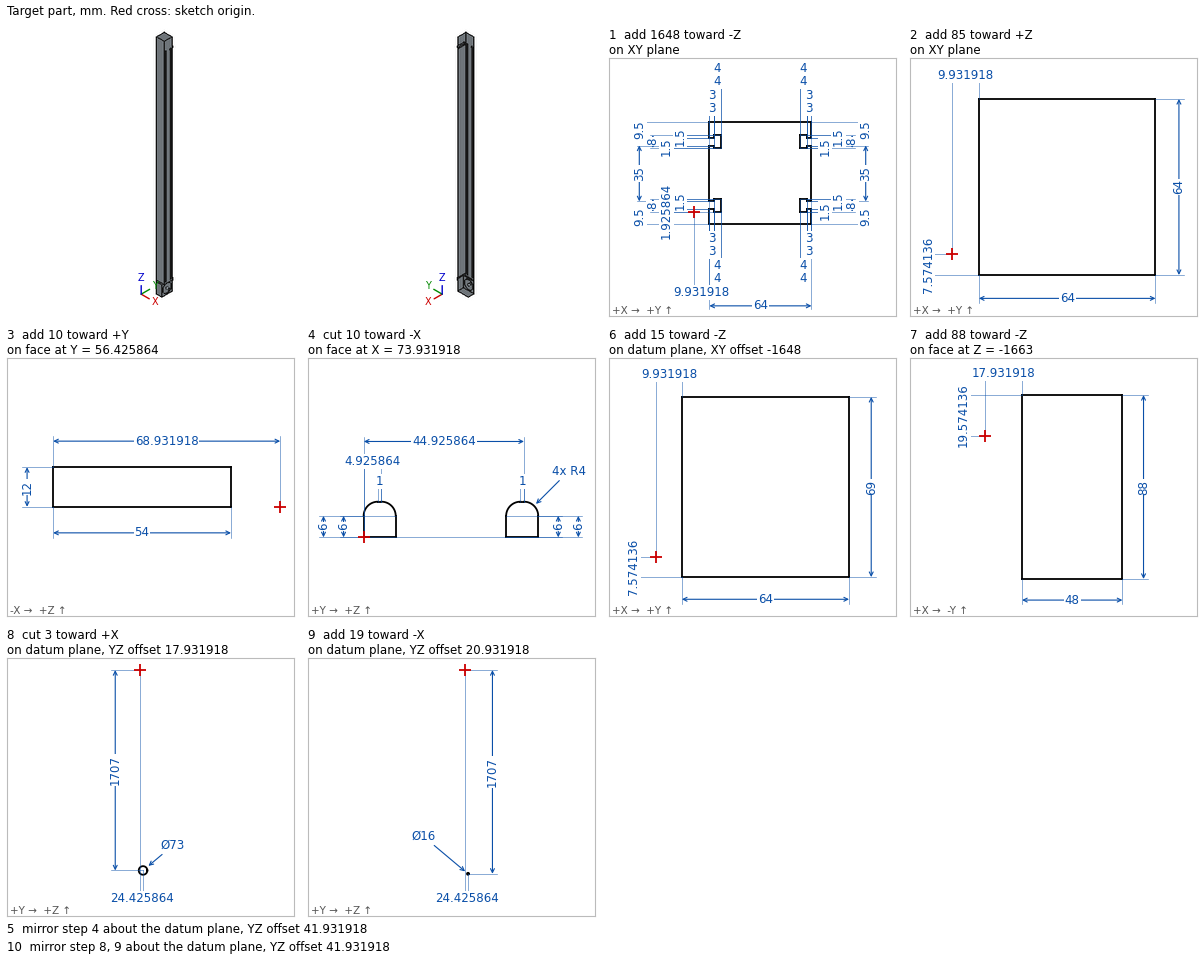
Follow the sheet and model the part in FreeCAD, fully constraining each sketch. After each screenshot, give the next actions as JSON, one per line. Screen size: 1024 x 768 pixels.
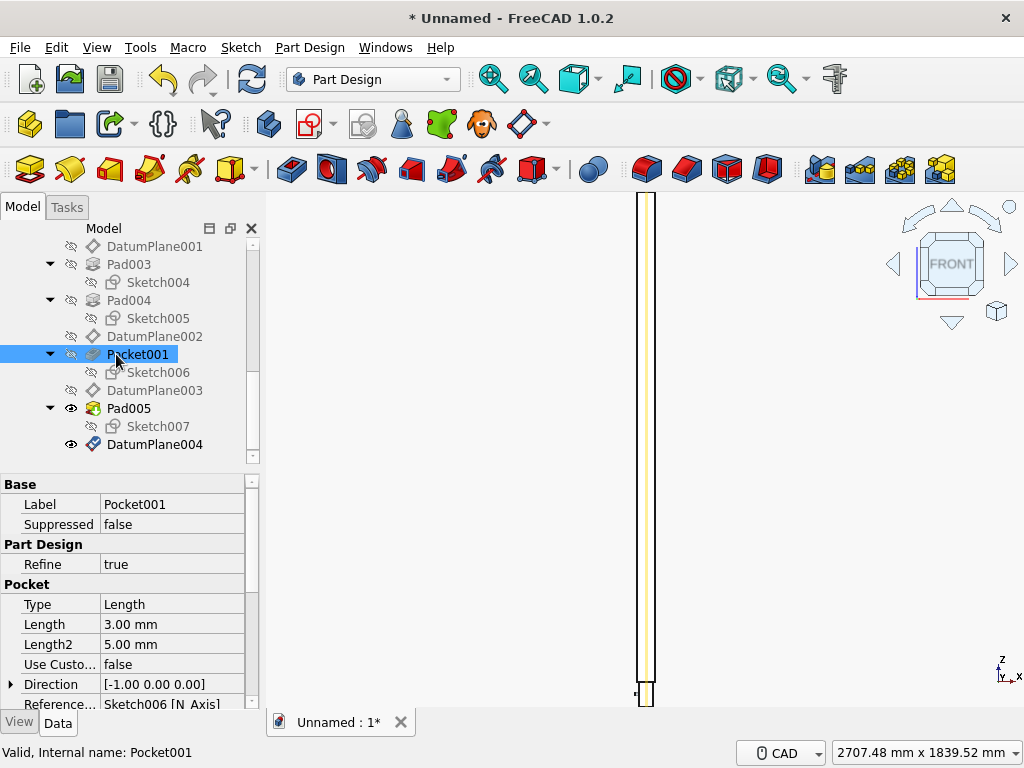
{"action": "left_click", "coordinate": [116, 408], "text": "ctrl"}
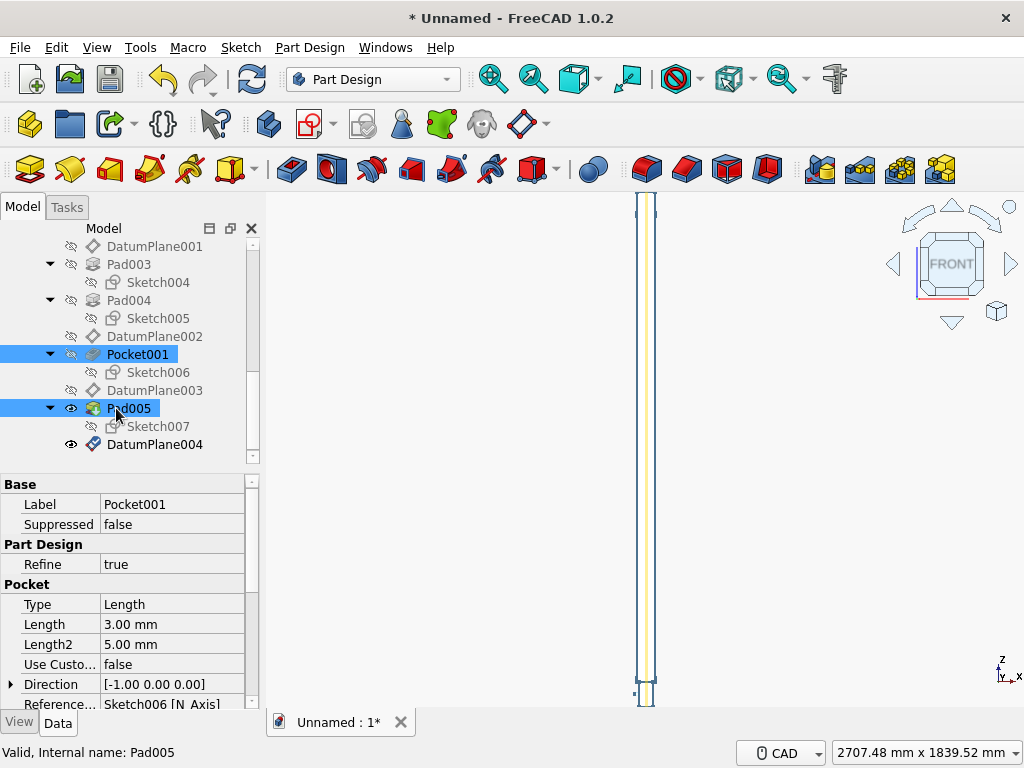
{"action": "left_click", "coordinate": [820, 170]}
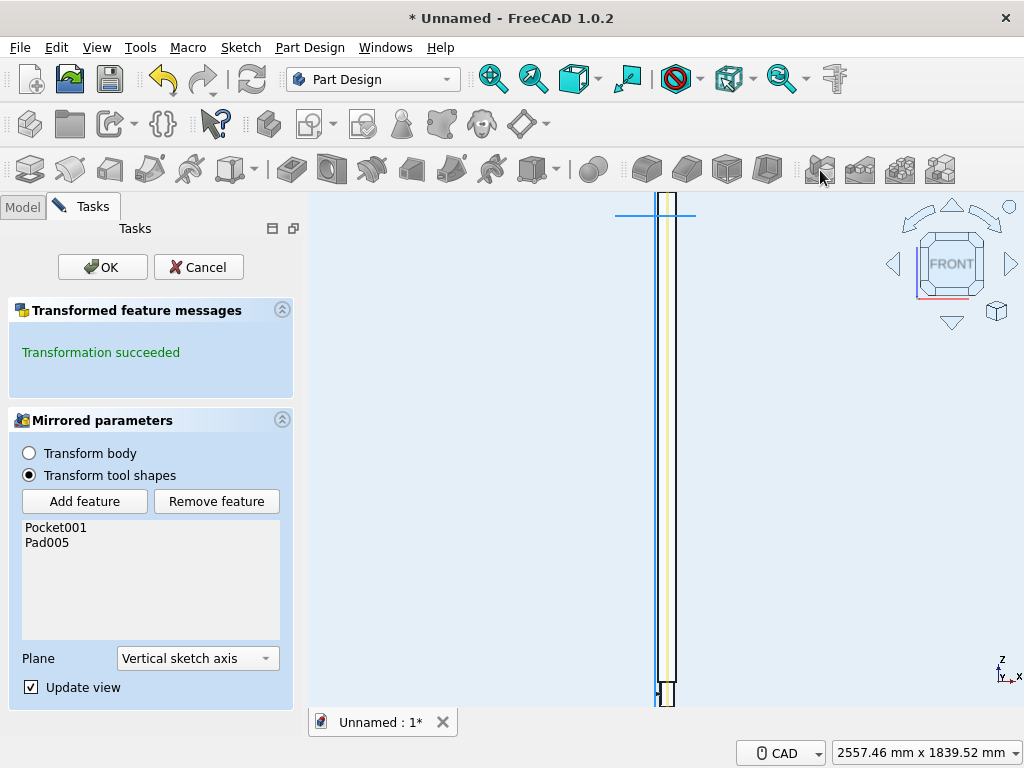
{"action": "left_click", "coordinate": [198, 658]}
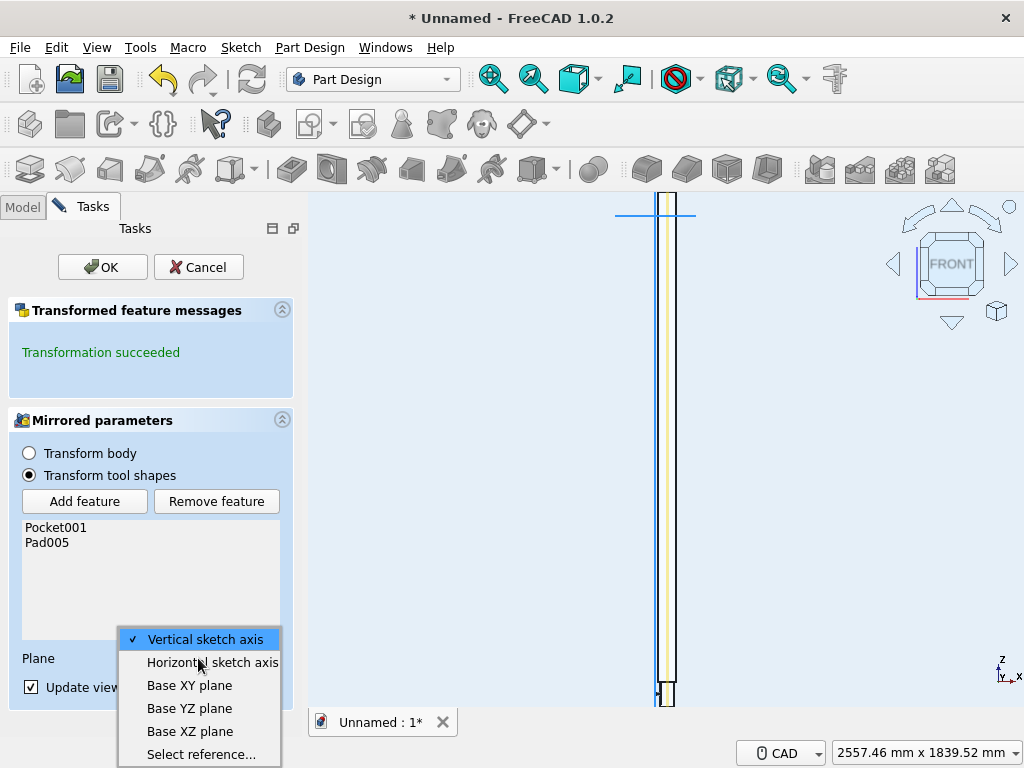
{"action": "left_click", "coordinate": [198, 754]}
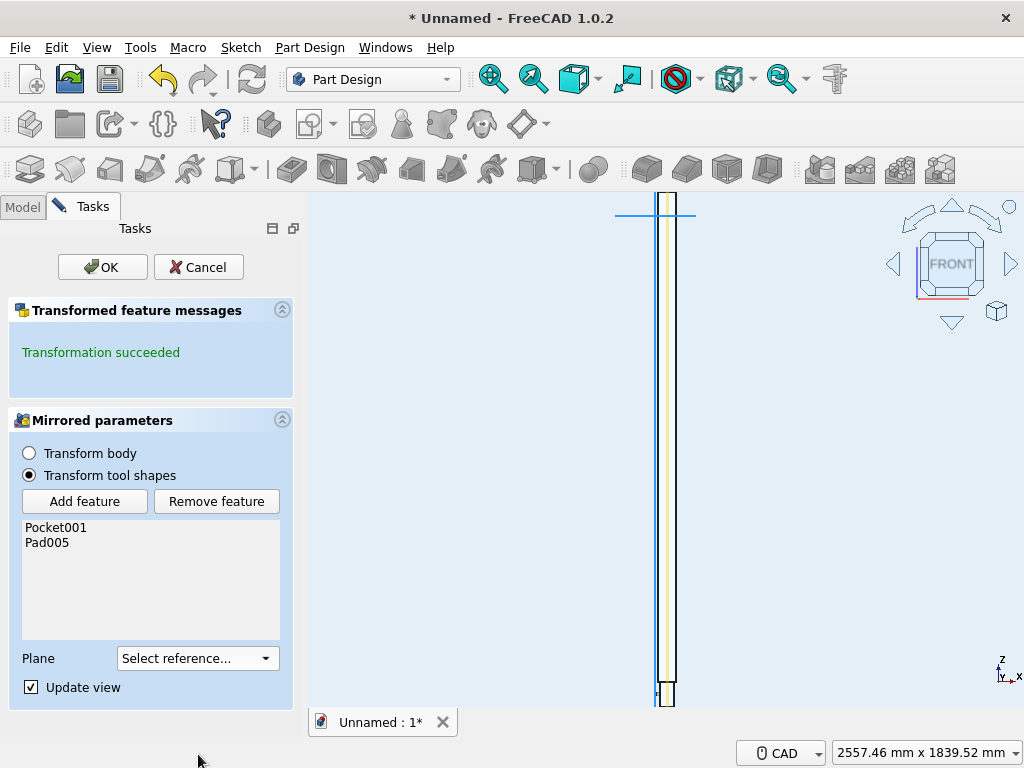
{"action": "left_click", "coordinate": [23, 206]}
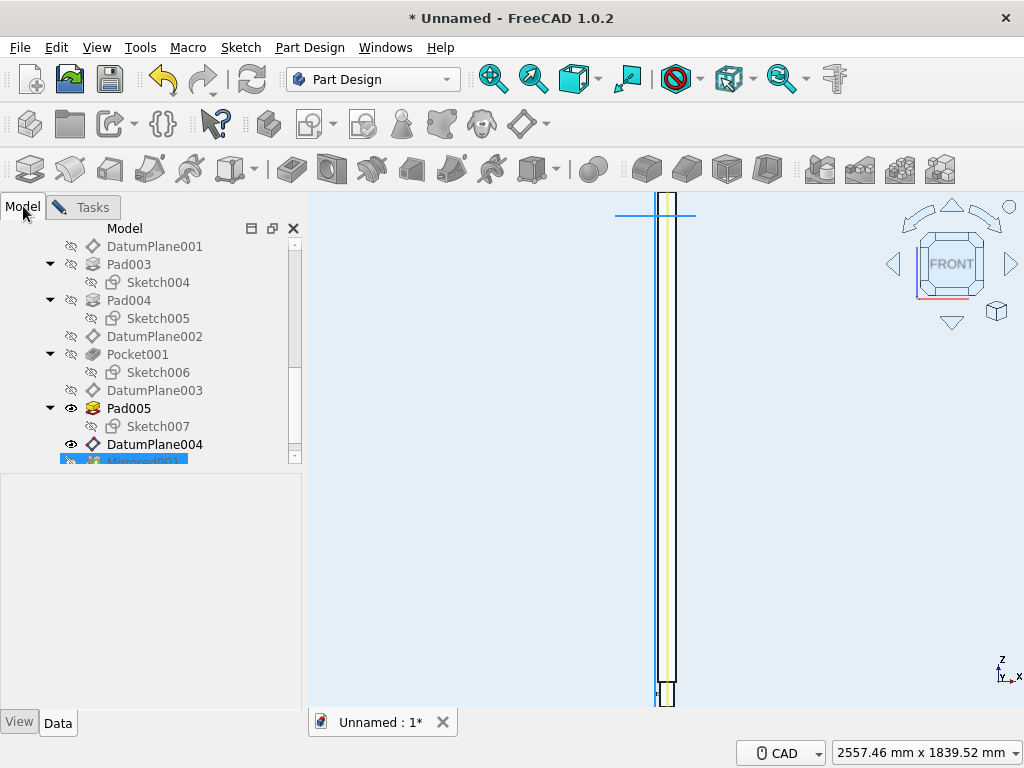
{"action": "left_click", "coordinate": [116, 444]}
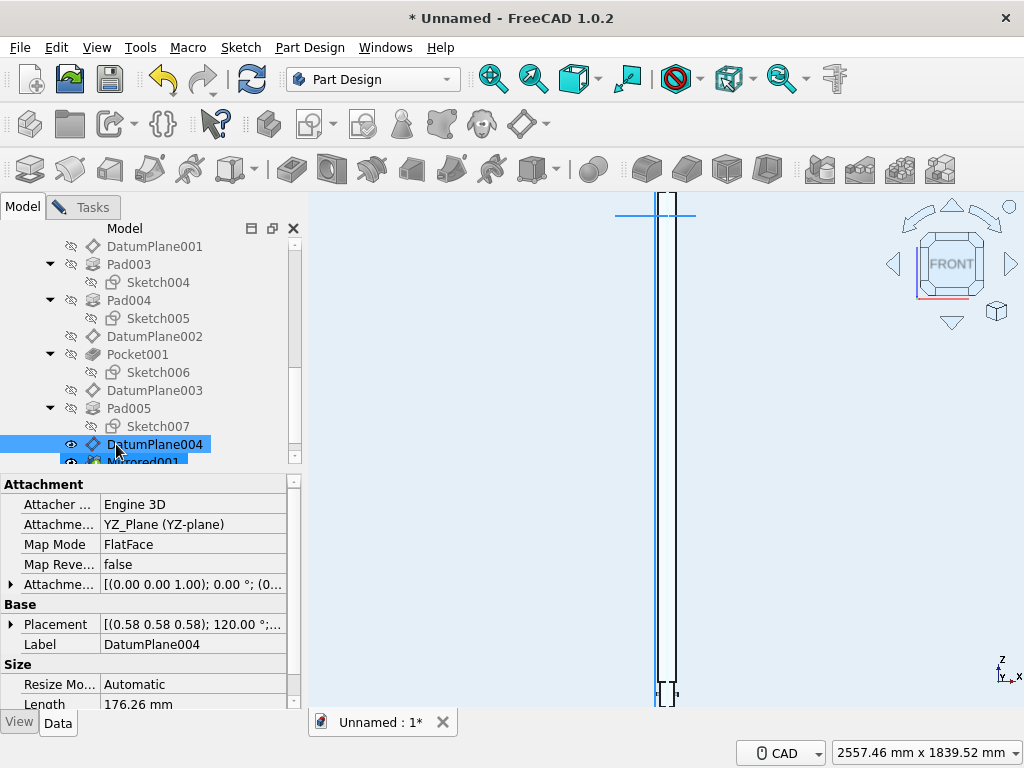
{"action": "left_click", "coordinate": [84, 206]}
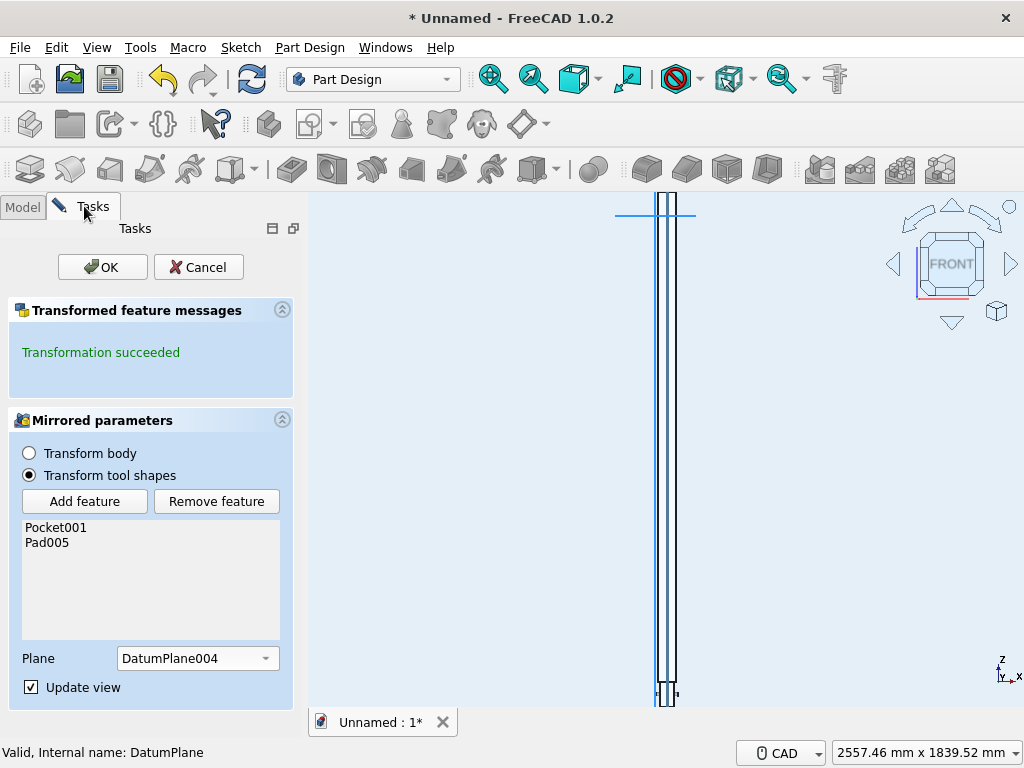
{"action": "left_click", "coordinate": [103, 267]}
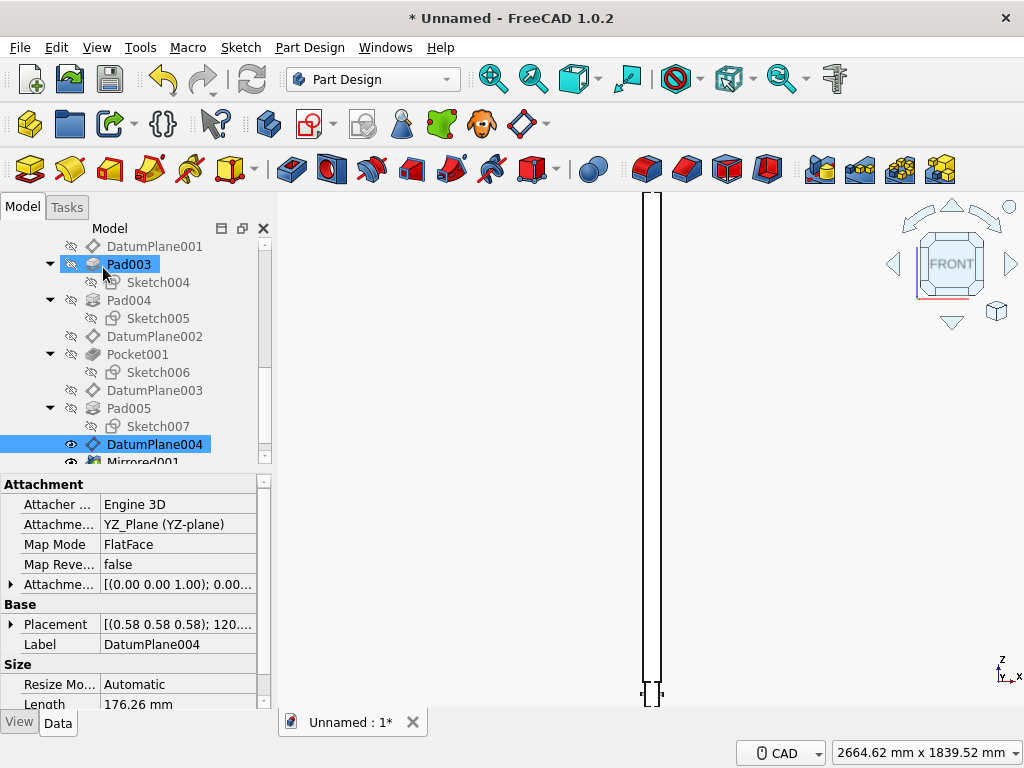
{"action": "left_click", "coordinate": [116, 444]}
{"action": "key", "text": "space"}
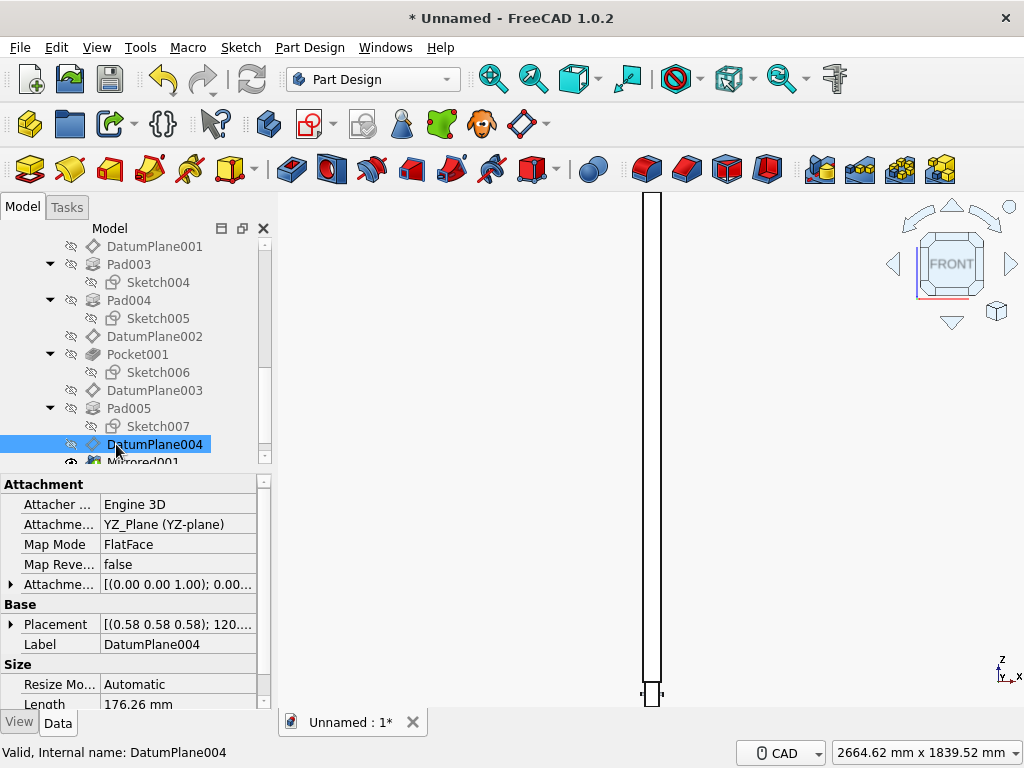
{"action": "key", "text": "0"}